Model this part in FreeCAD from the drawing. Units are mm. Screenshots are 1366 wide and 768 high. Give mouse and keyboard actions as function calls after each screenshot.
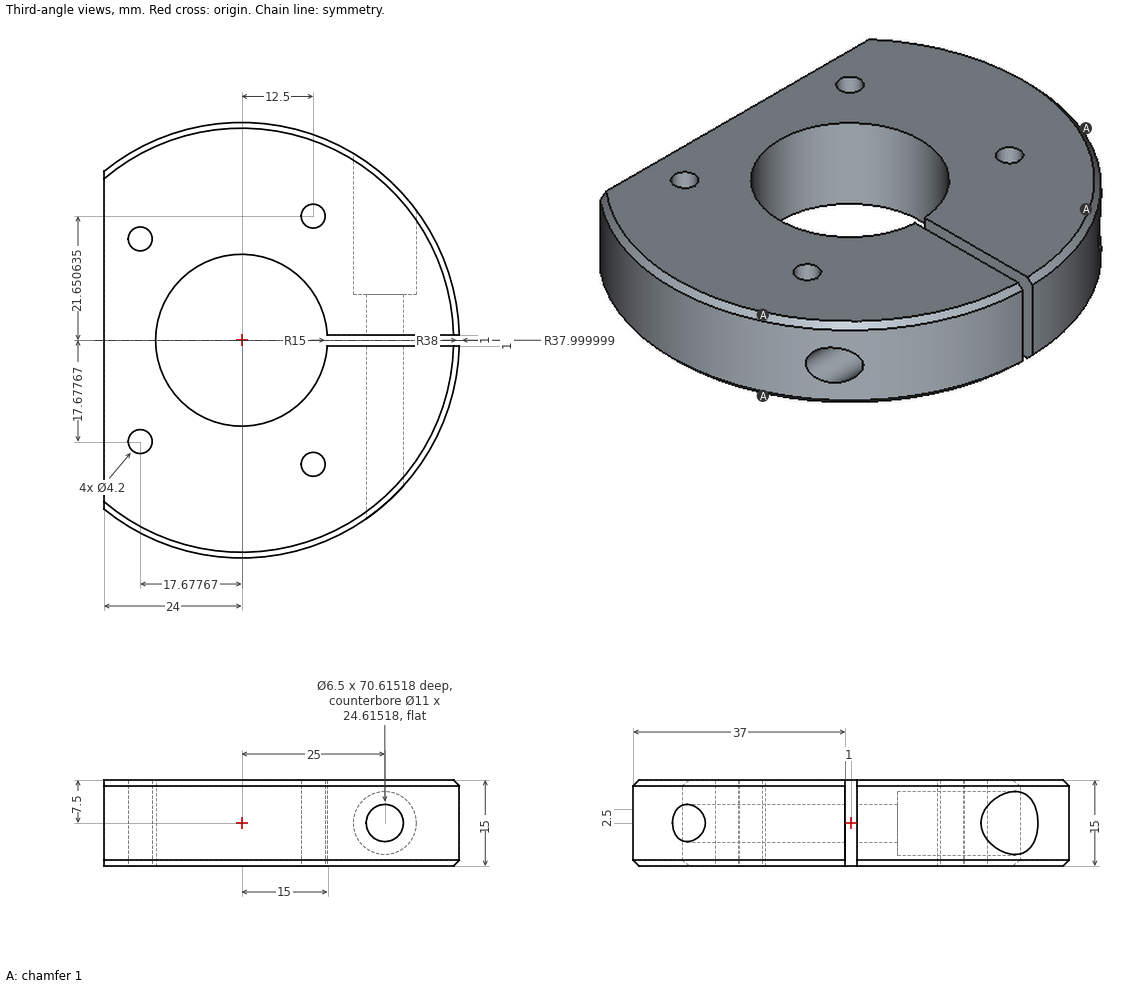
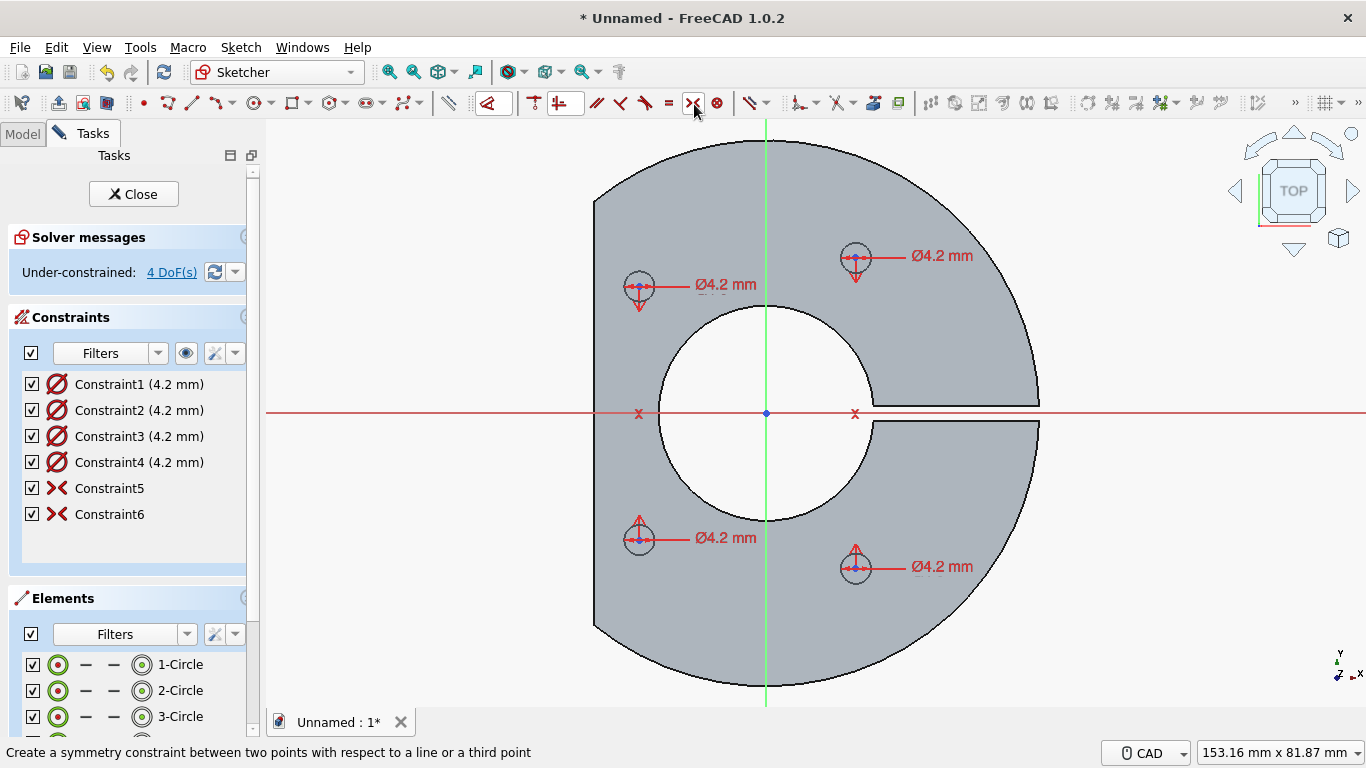
click(856, 258)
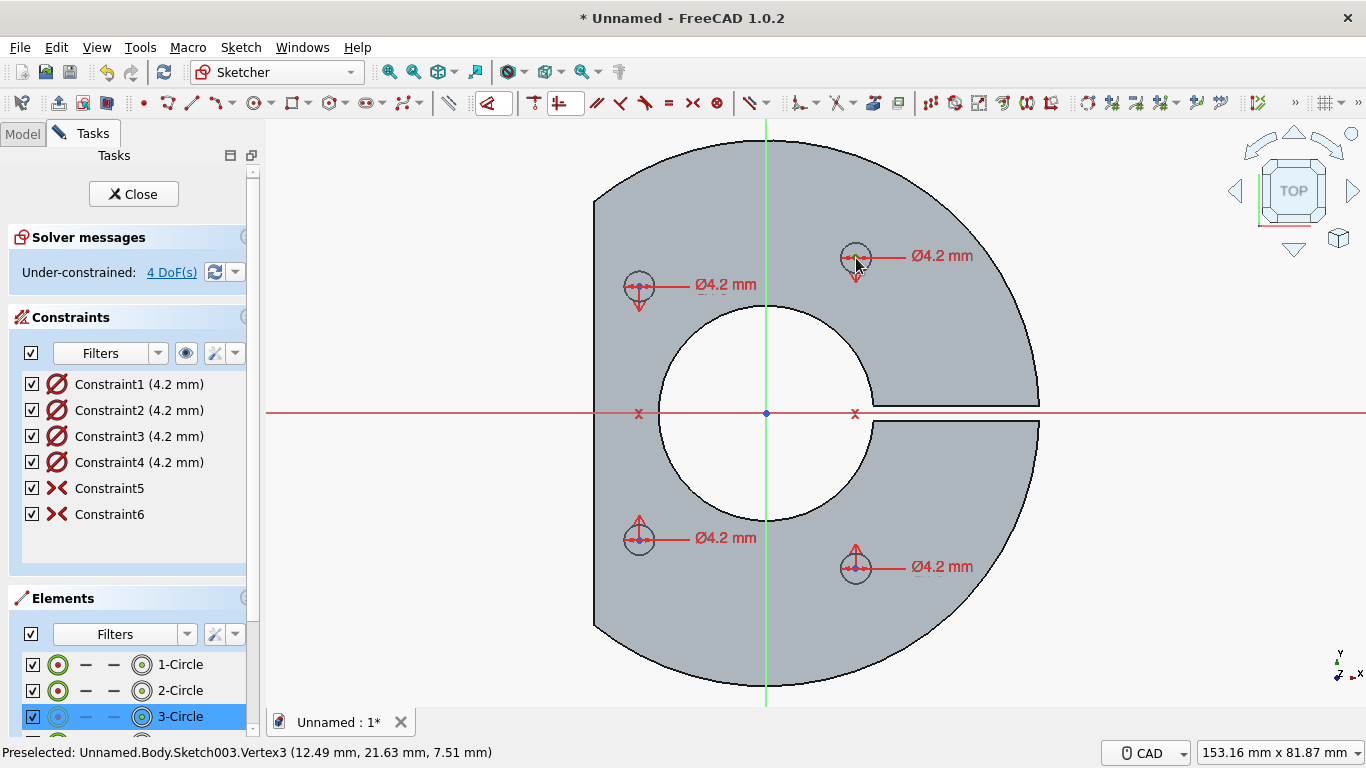
key(l)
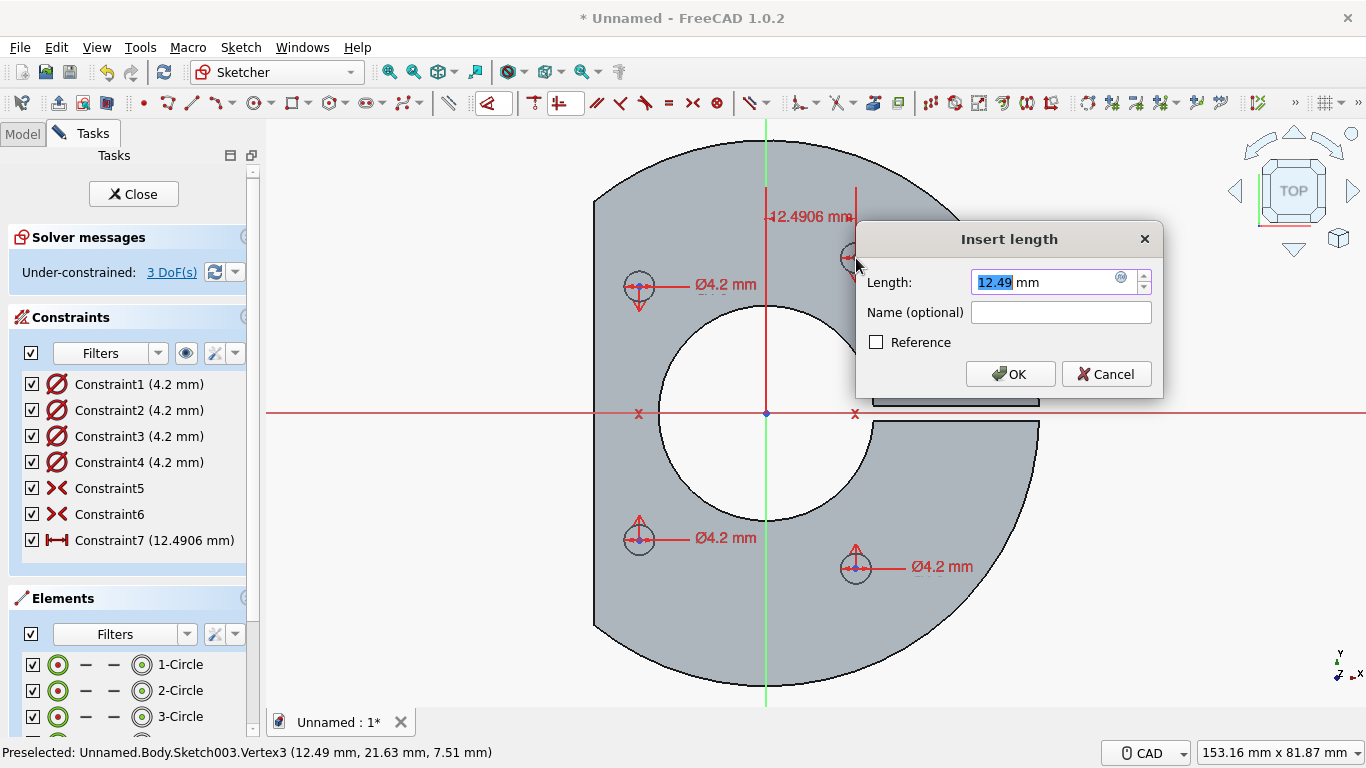
text(12.5)
key(Return)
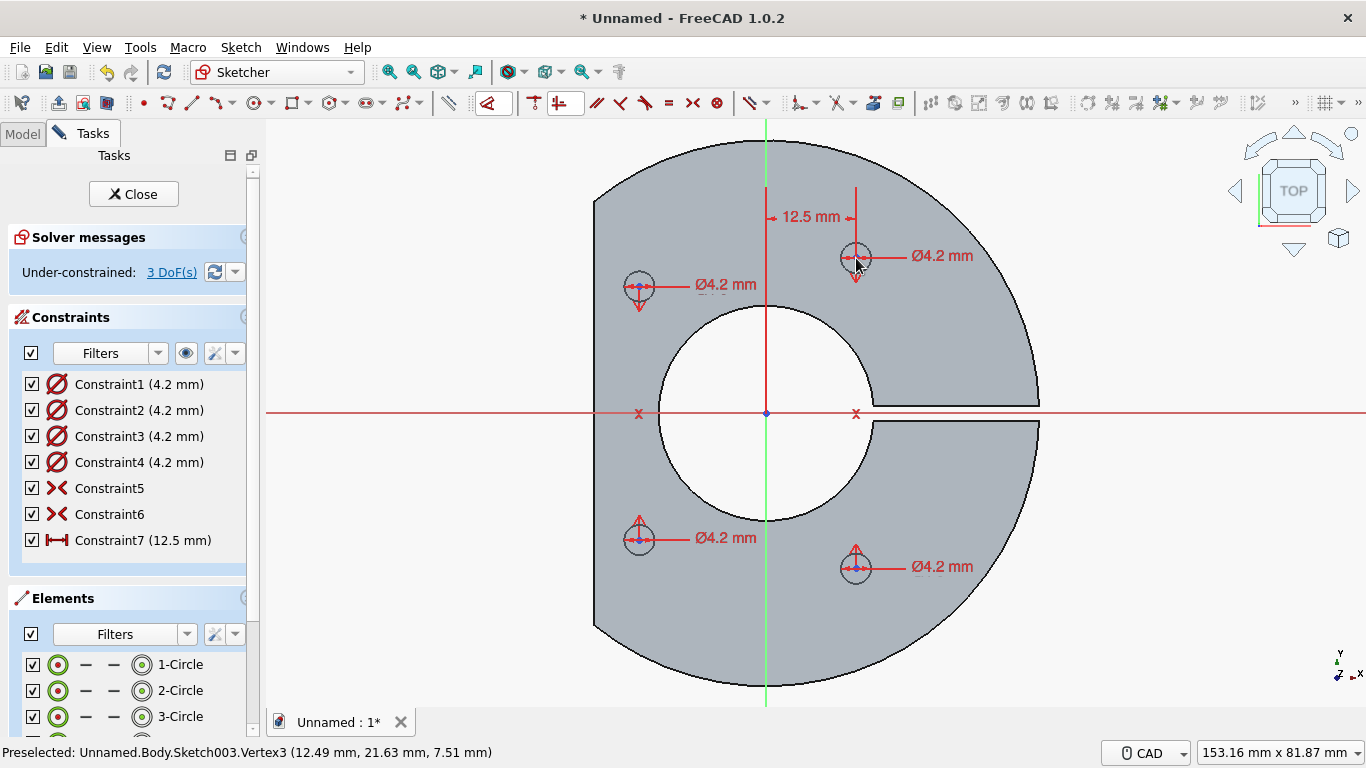
click(639, 540)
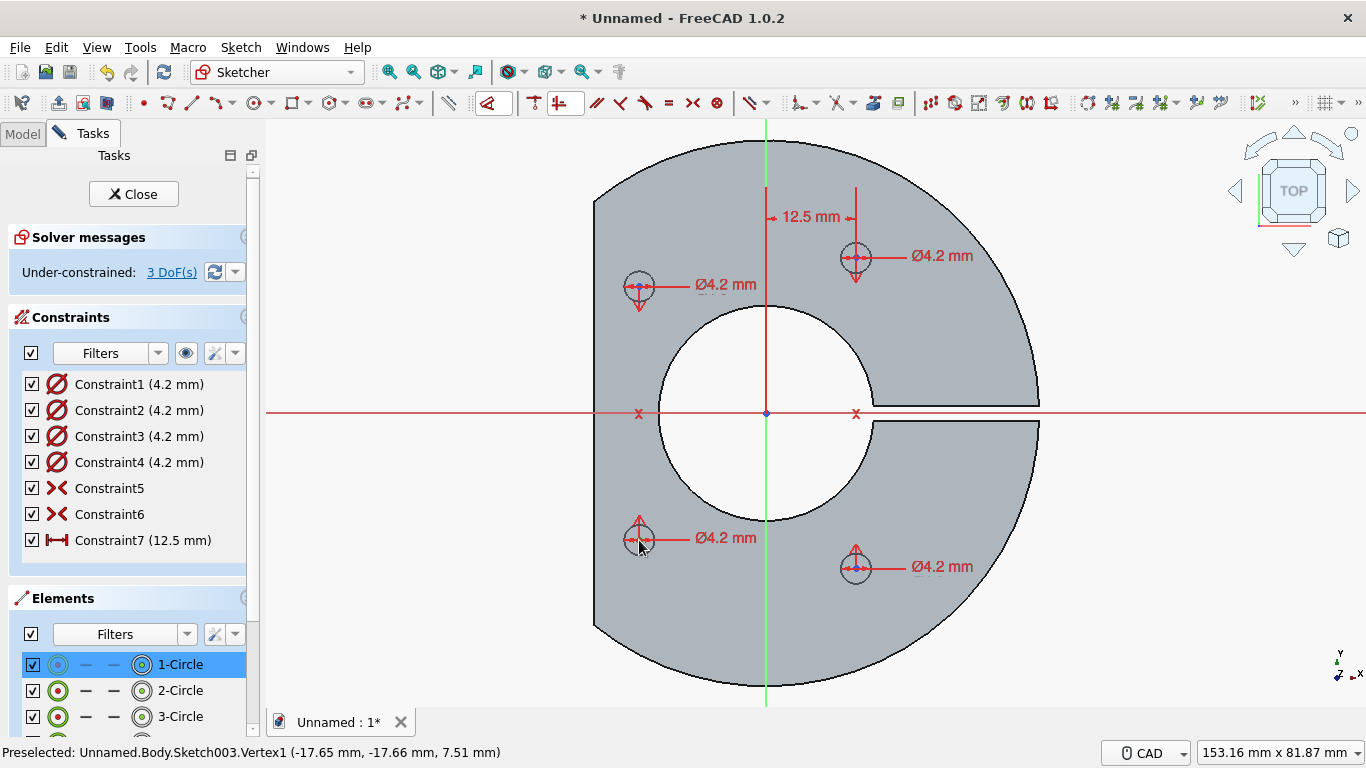
key(l)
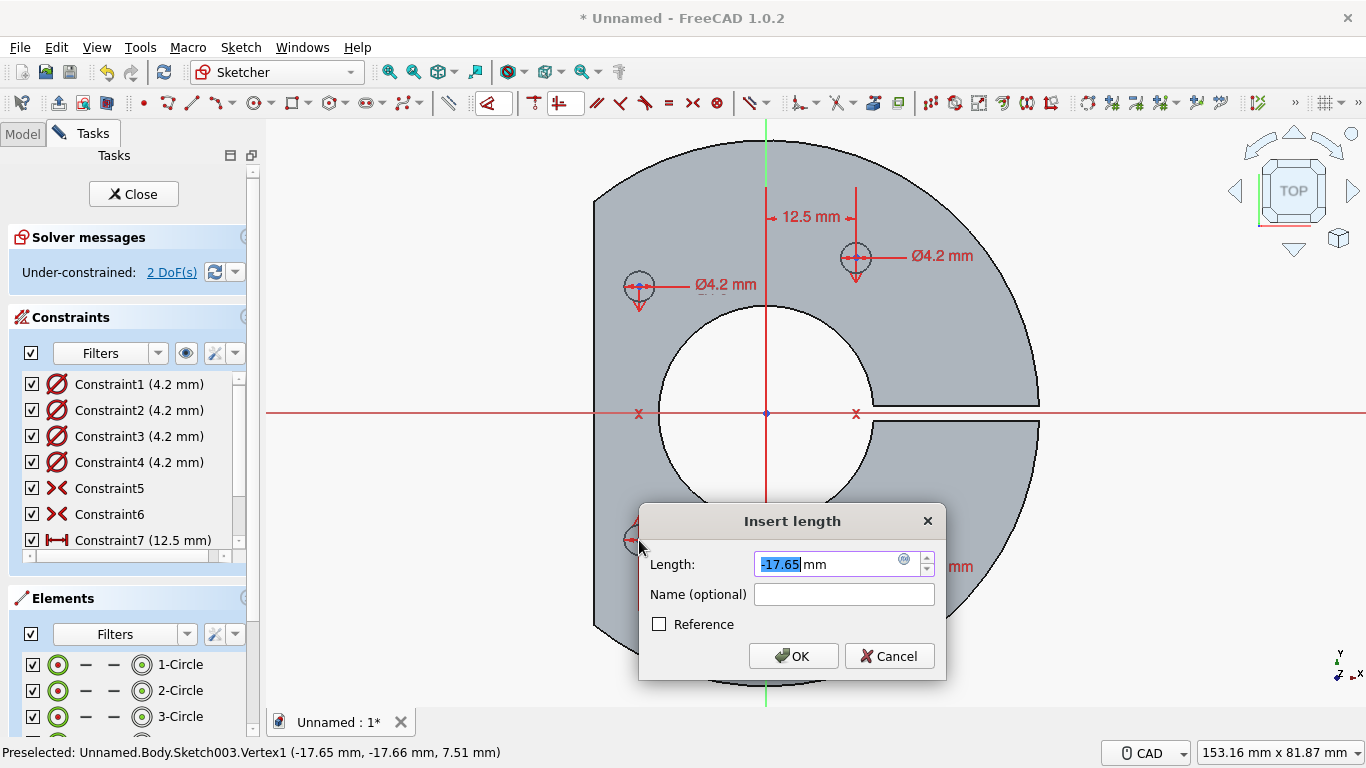
text(-17.67767)
key(Return)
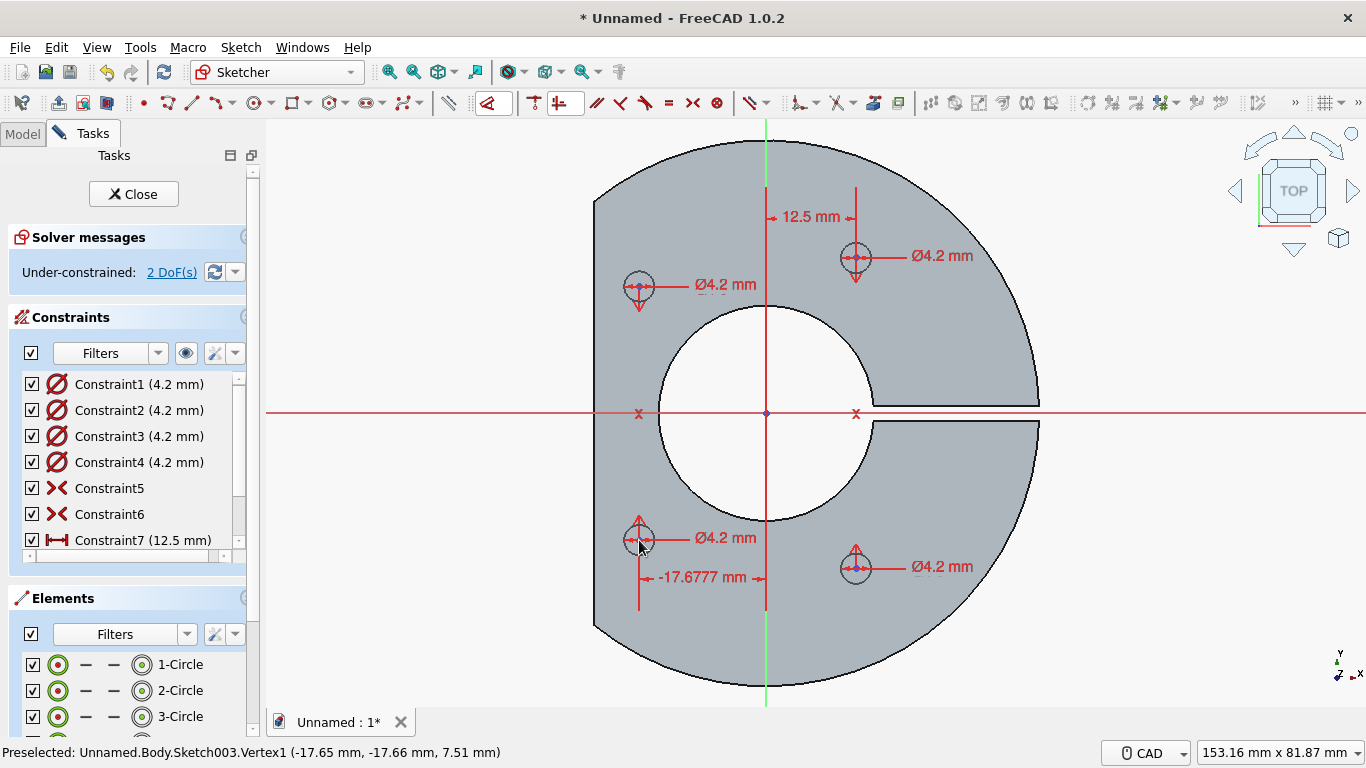
click(639, 540)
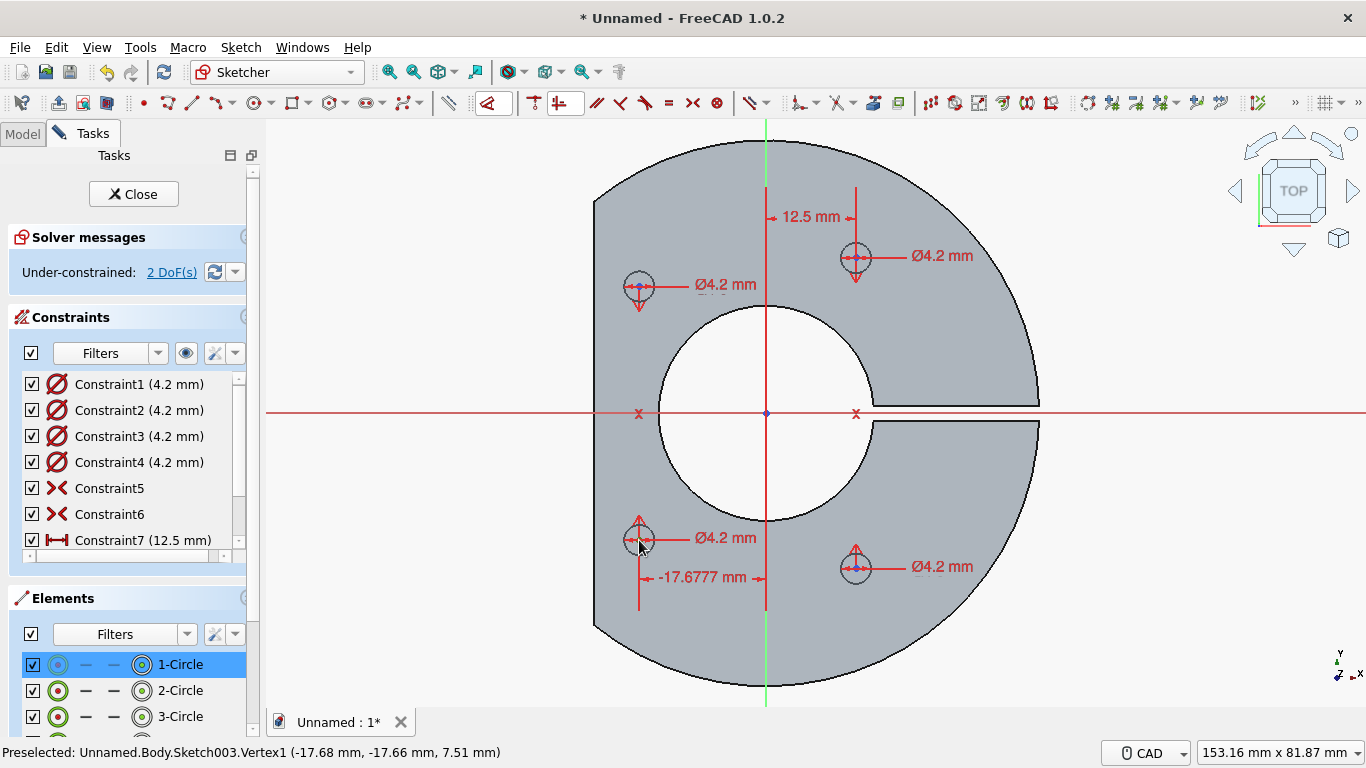
key(i)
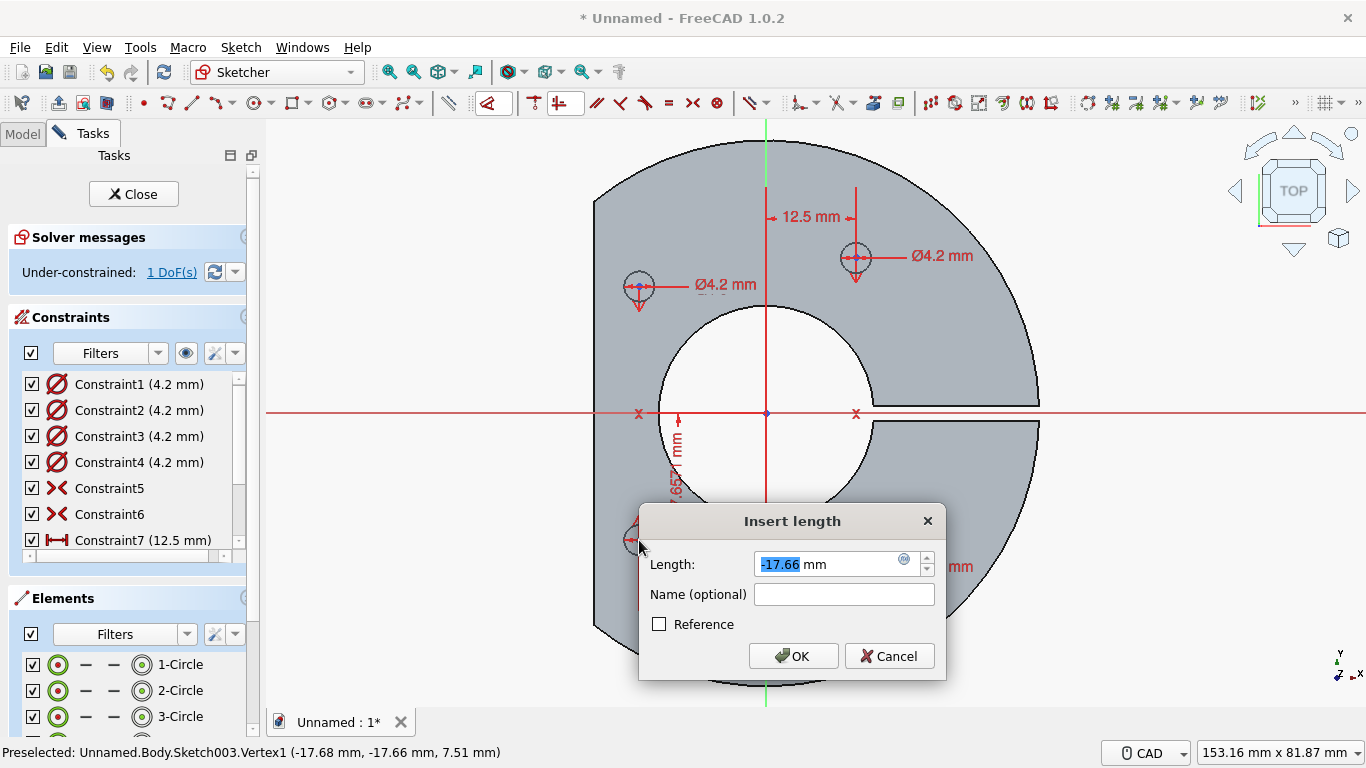
text(-17.67767)
key(Return)